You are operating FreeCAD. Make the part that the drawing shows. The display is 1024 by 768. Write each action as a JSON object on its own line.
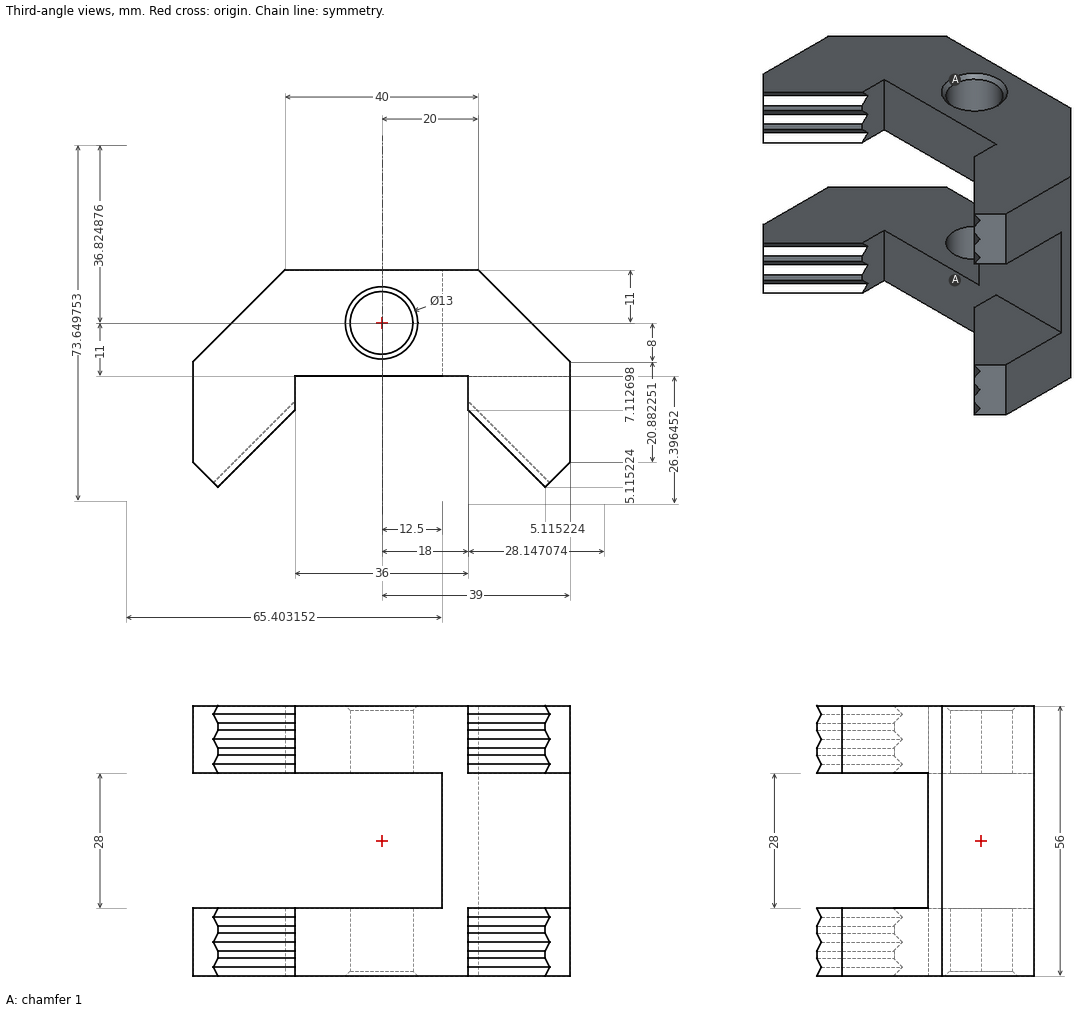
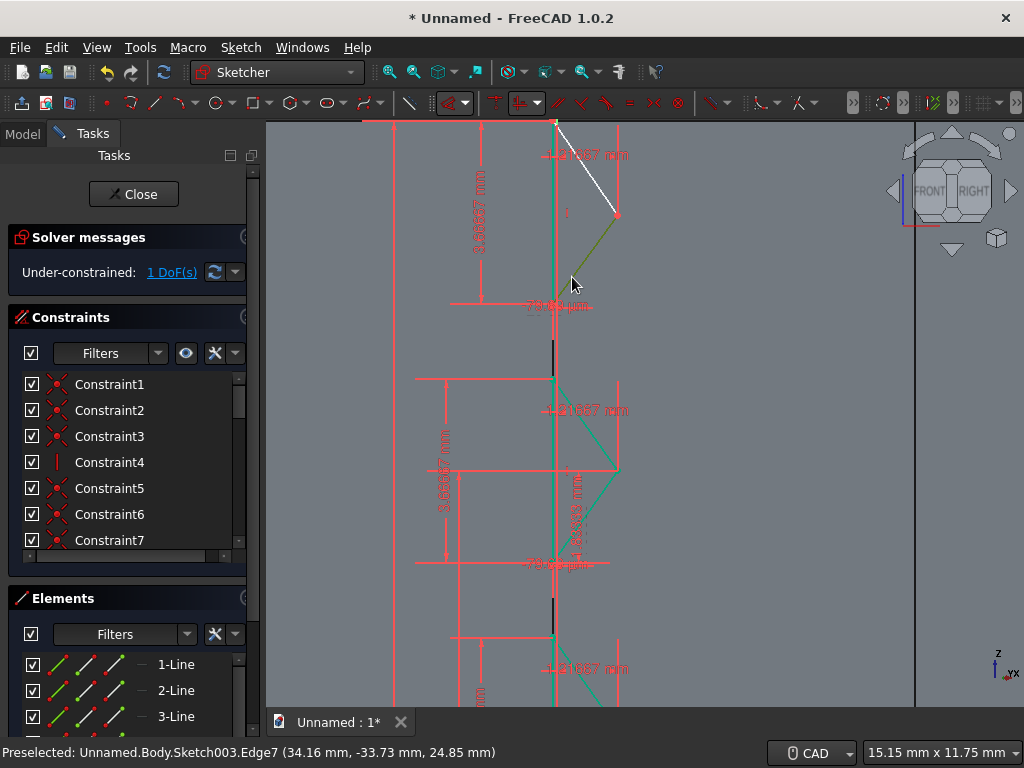
{"action": "left_click", "coordinate": [468, 104]}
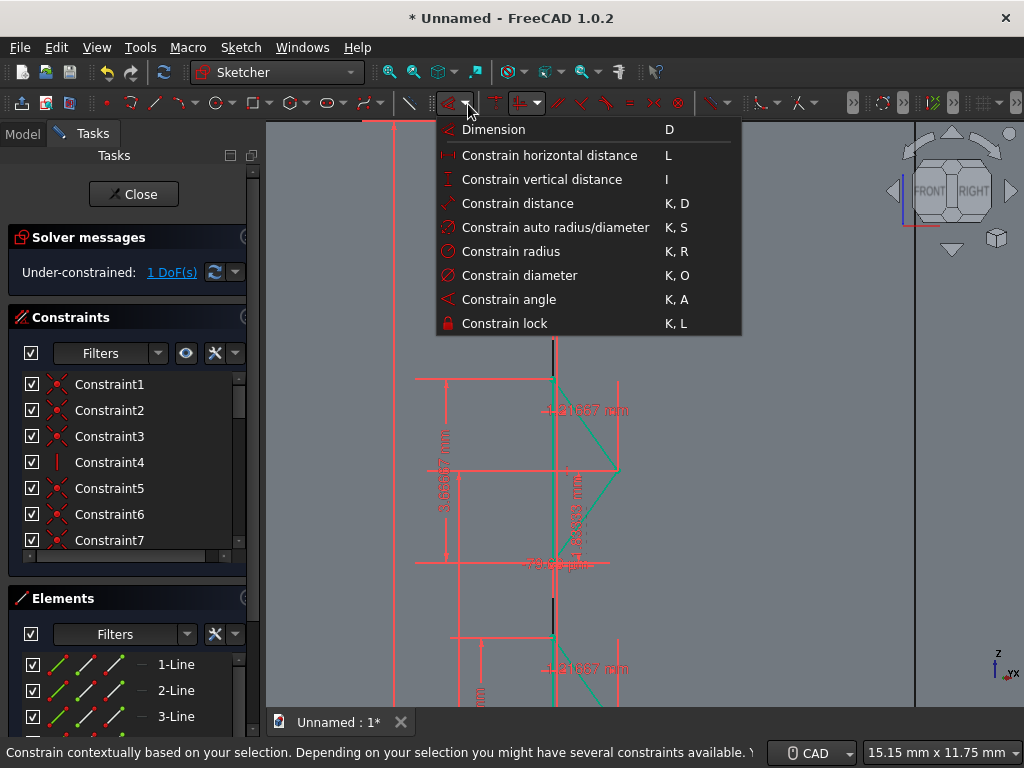
{"action": "left_click", "coordinate": [589, 179]}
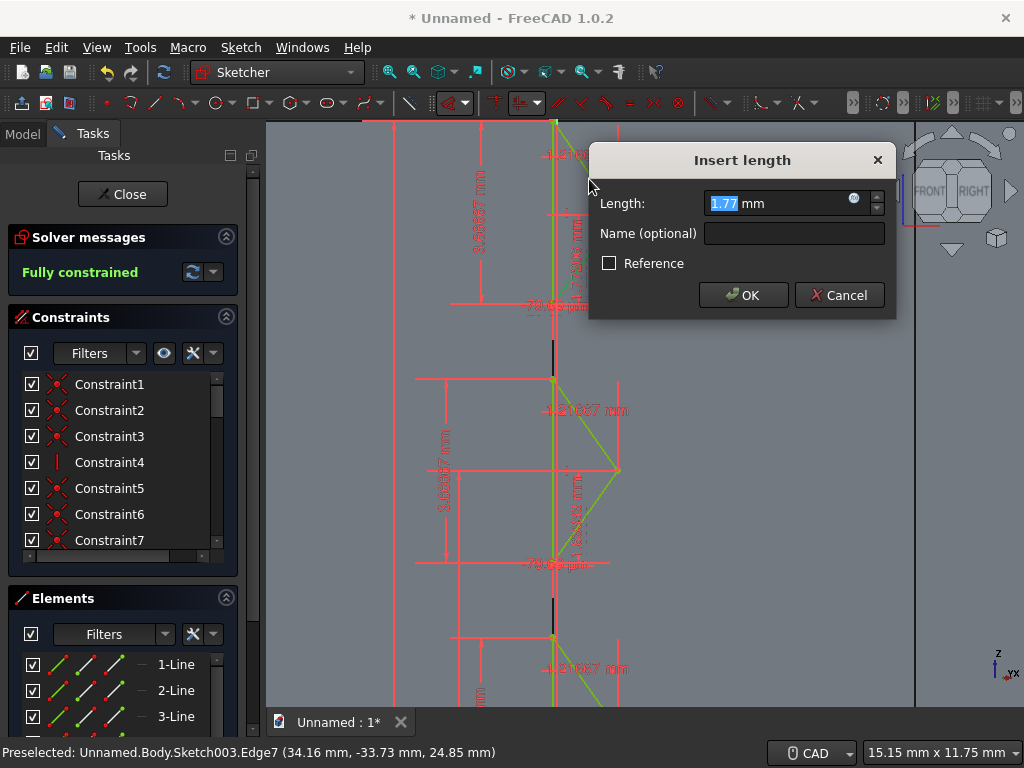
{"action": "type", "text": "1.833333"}
{"action": "key", "text": "Return"}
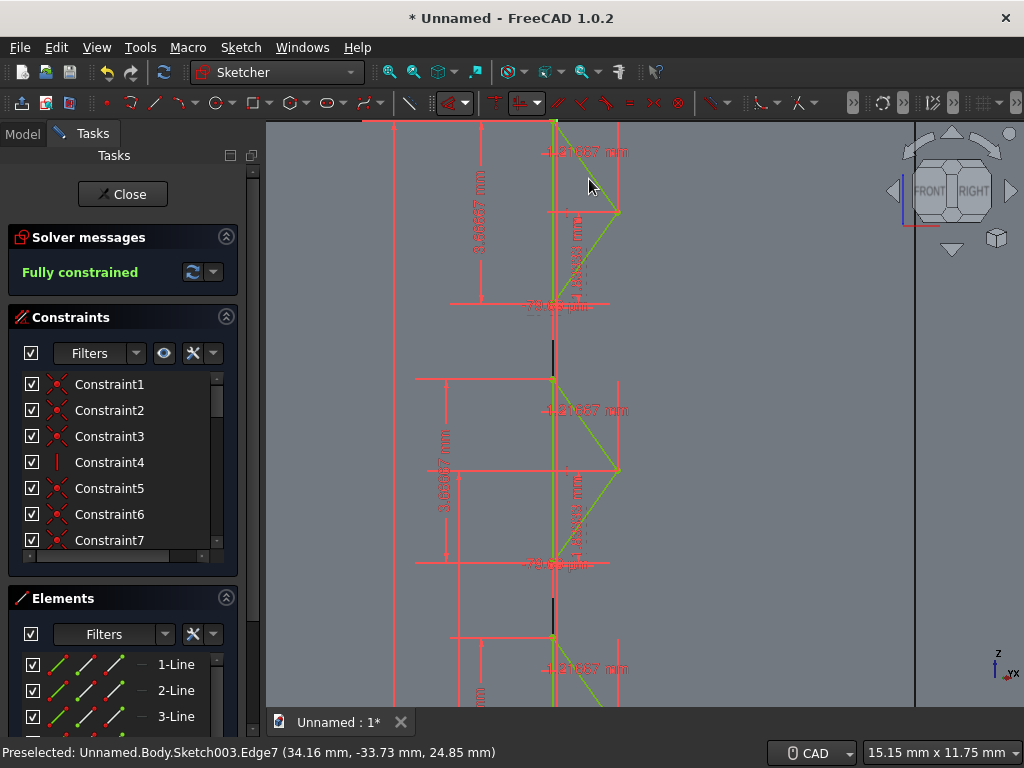
{"action": "left_click", "coordinate": [123, 194]}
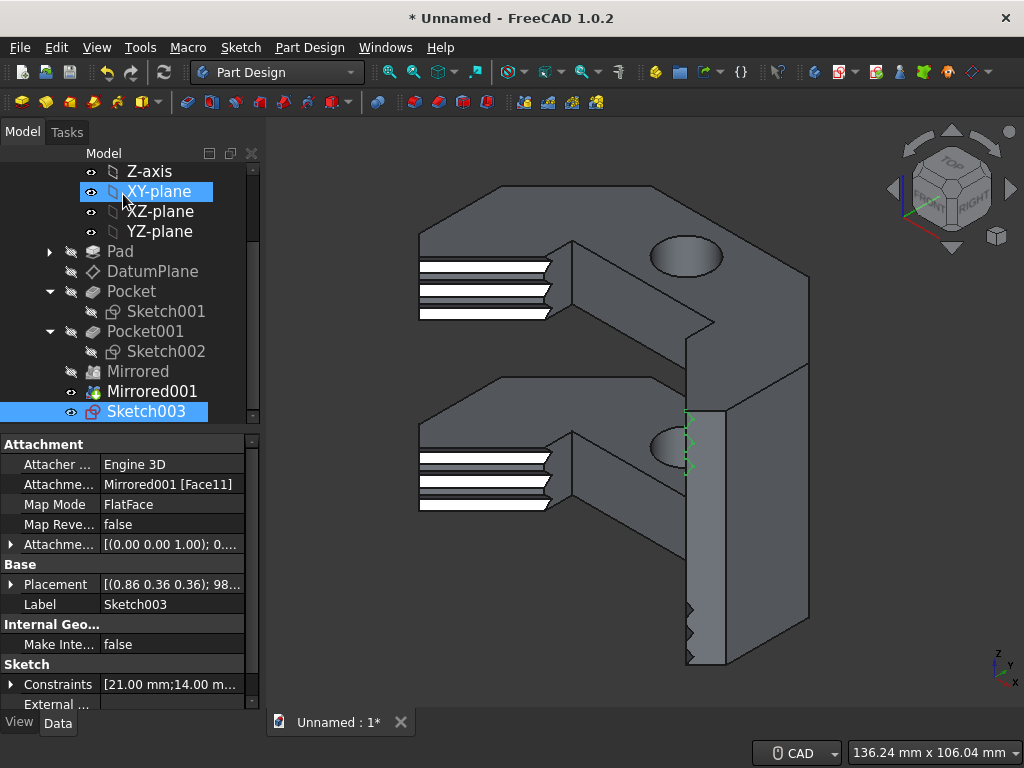
{"action": "left_click", "coordinate": [188, 102]}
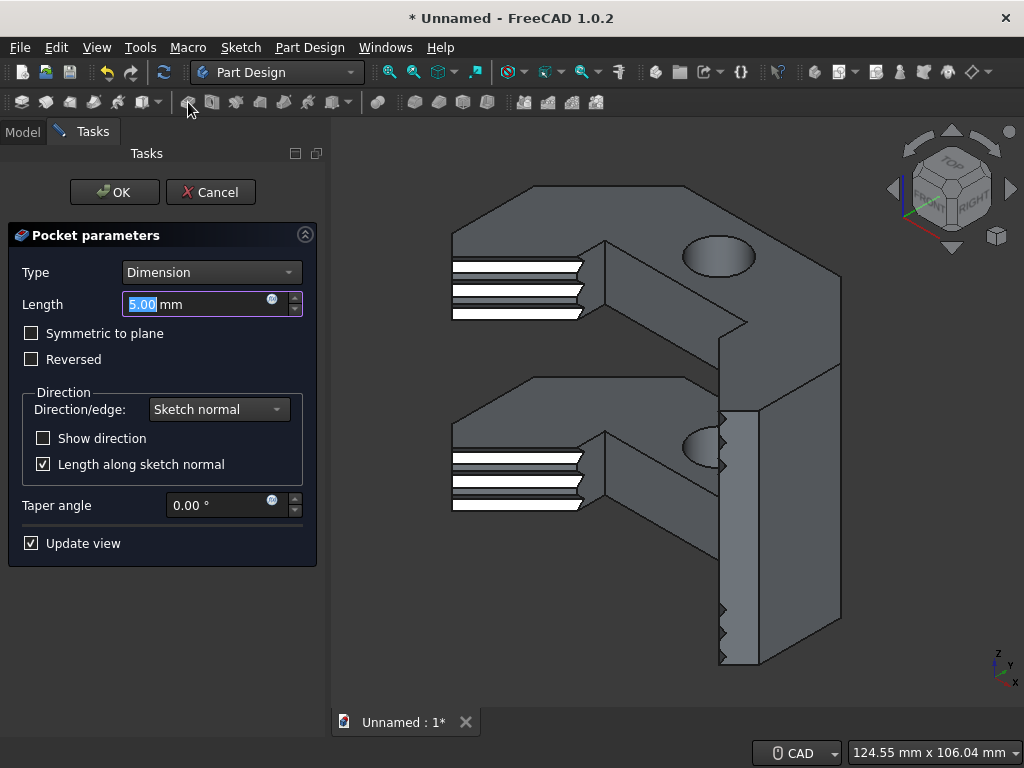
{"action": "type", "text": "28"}
{"action": "key", "text": "Tab"}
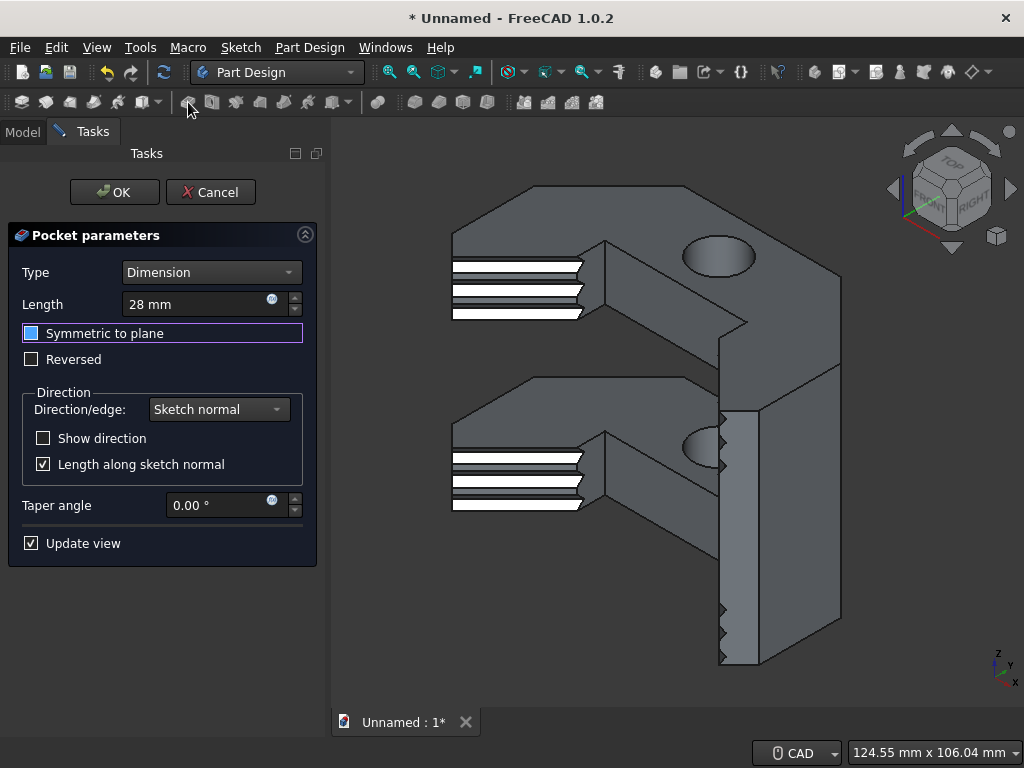
{"action": "left_click", "coordinate": [115, 192]}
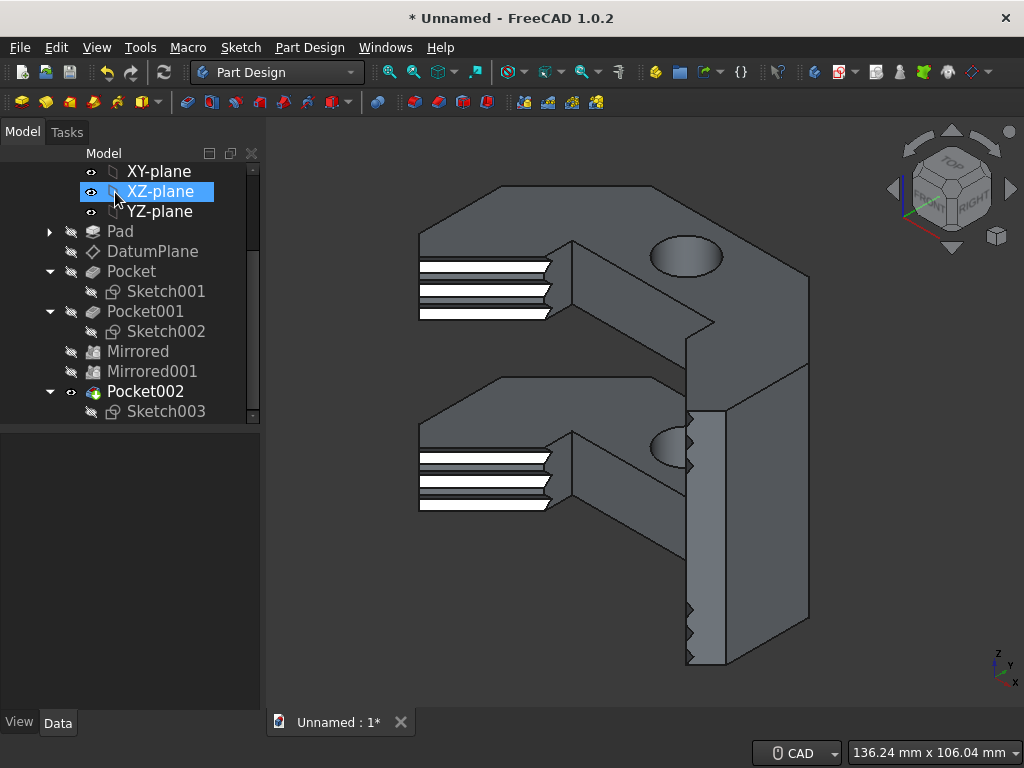
{"action": "left_click", "coordinate": [661, 241]}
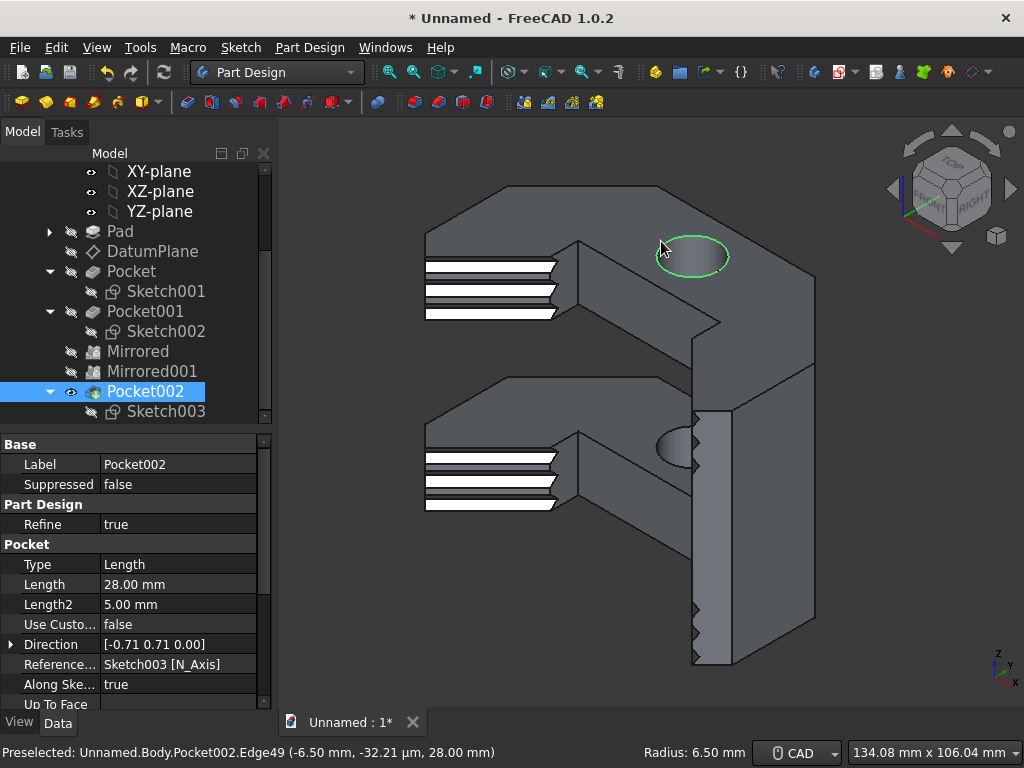
{"action": "key", "text": "2"}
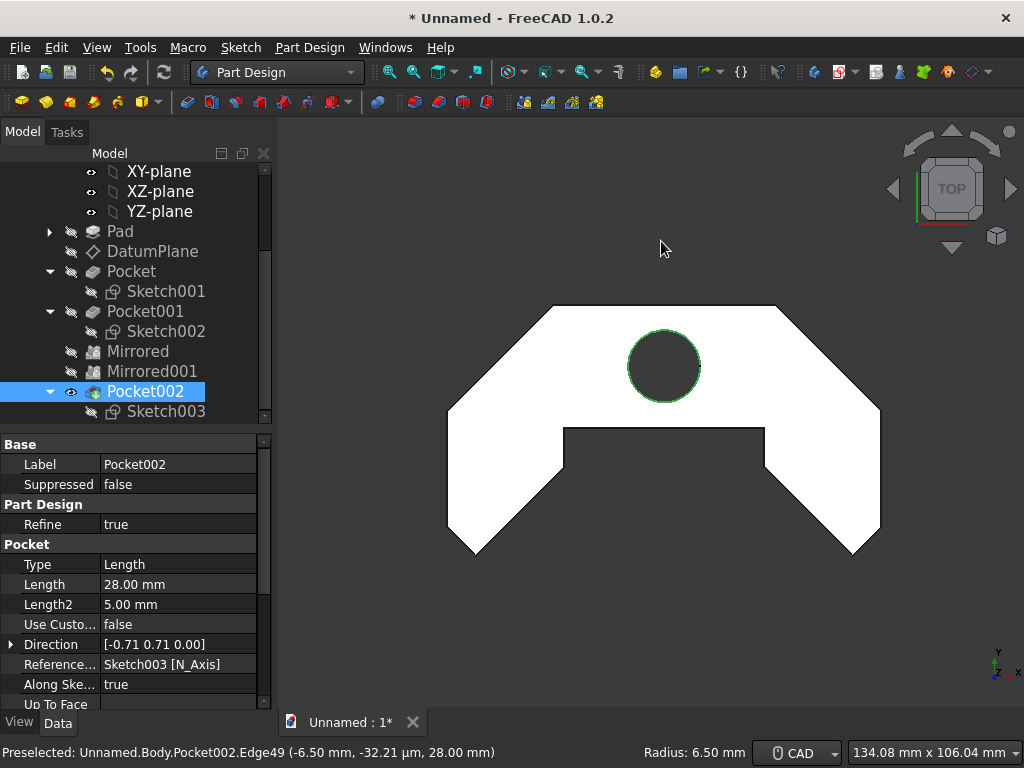
{"action": "key", "text": "0"}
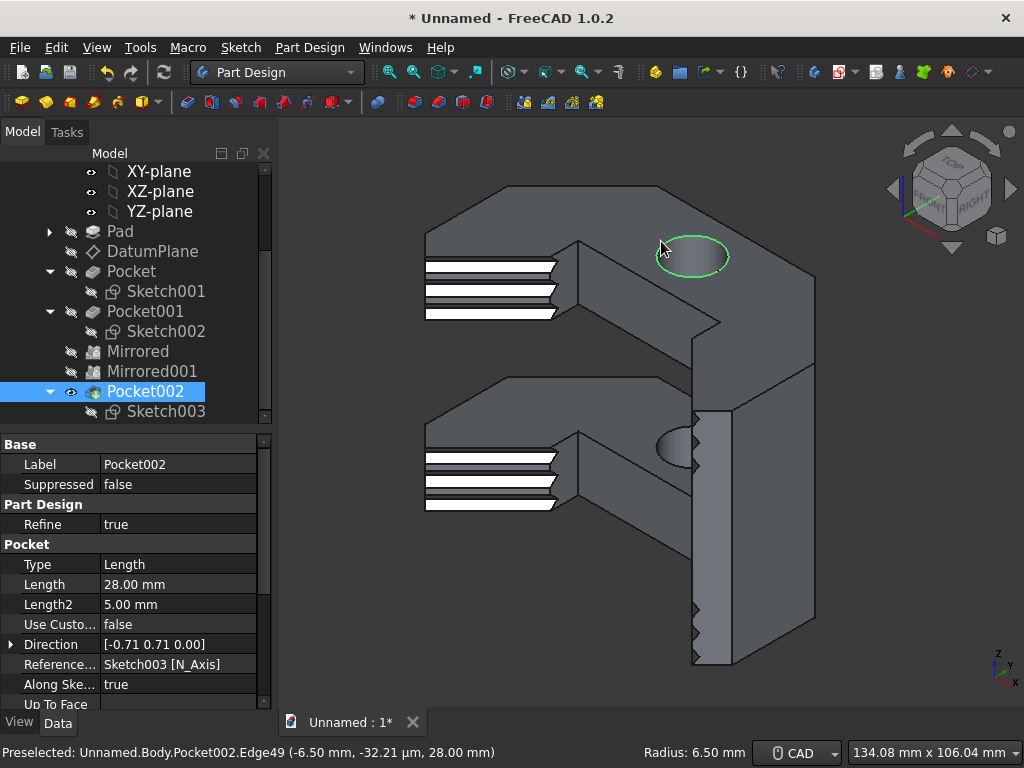
{"action": "key", "text": "1"}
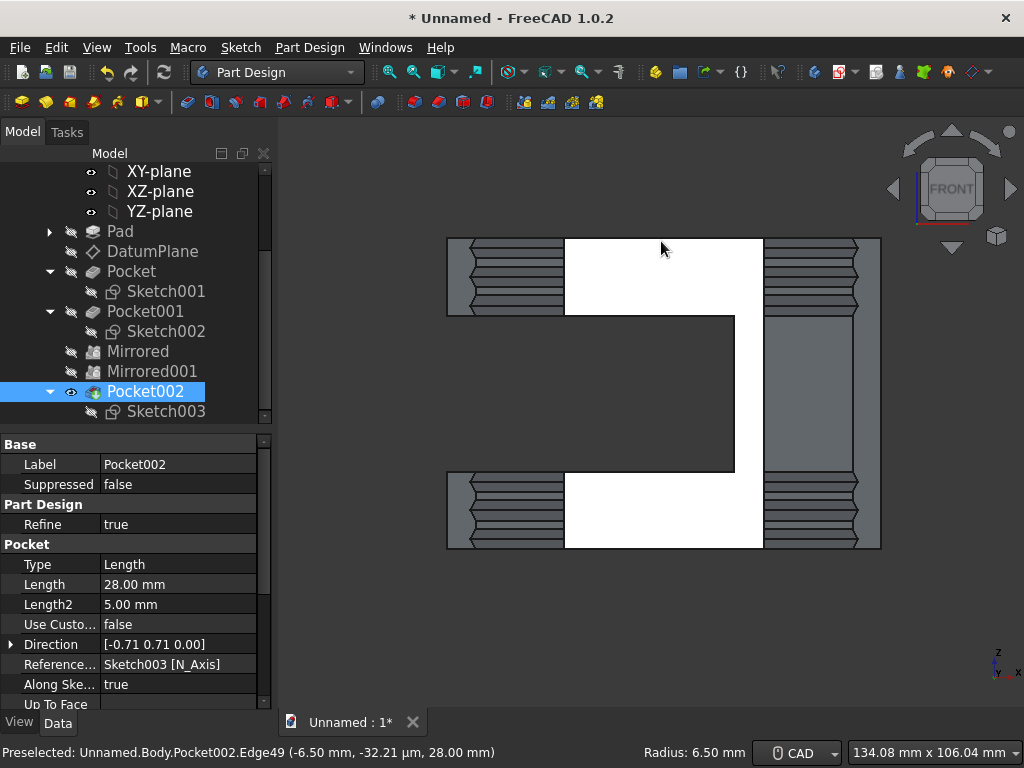
{"action": "key", "text": "3"}